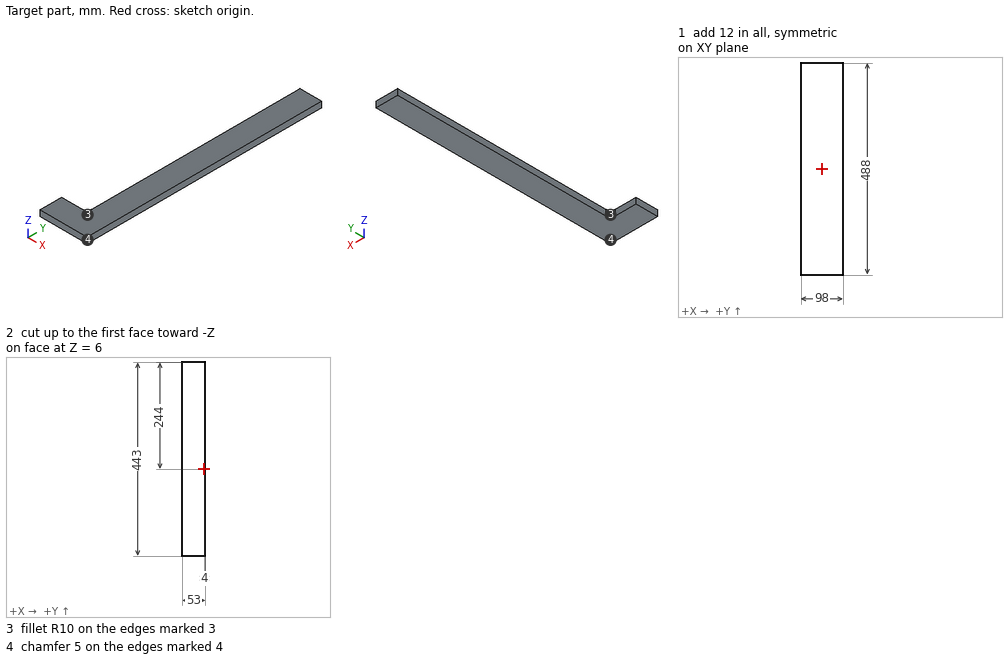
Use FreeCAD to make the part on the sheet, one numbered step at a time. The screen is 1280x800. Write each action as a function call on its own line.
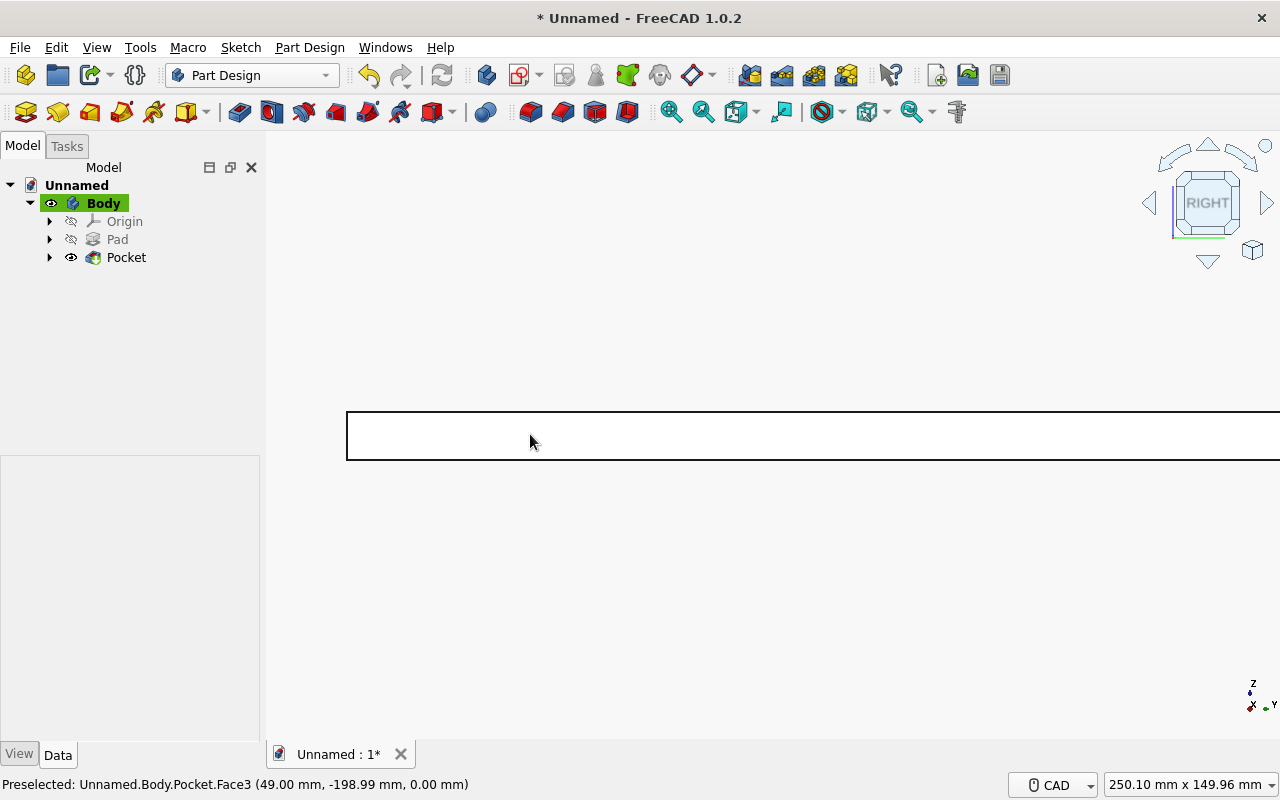
key(v)
key(f)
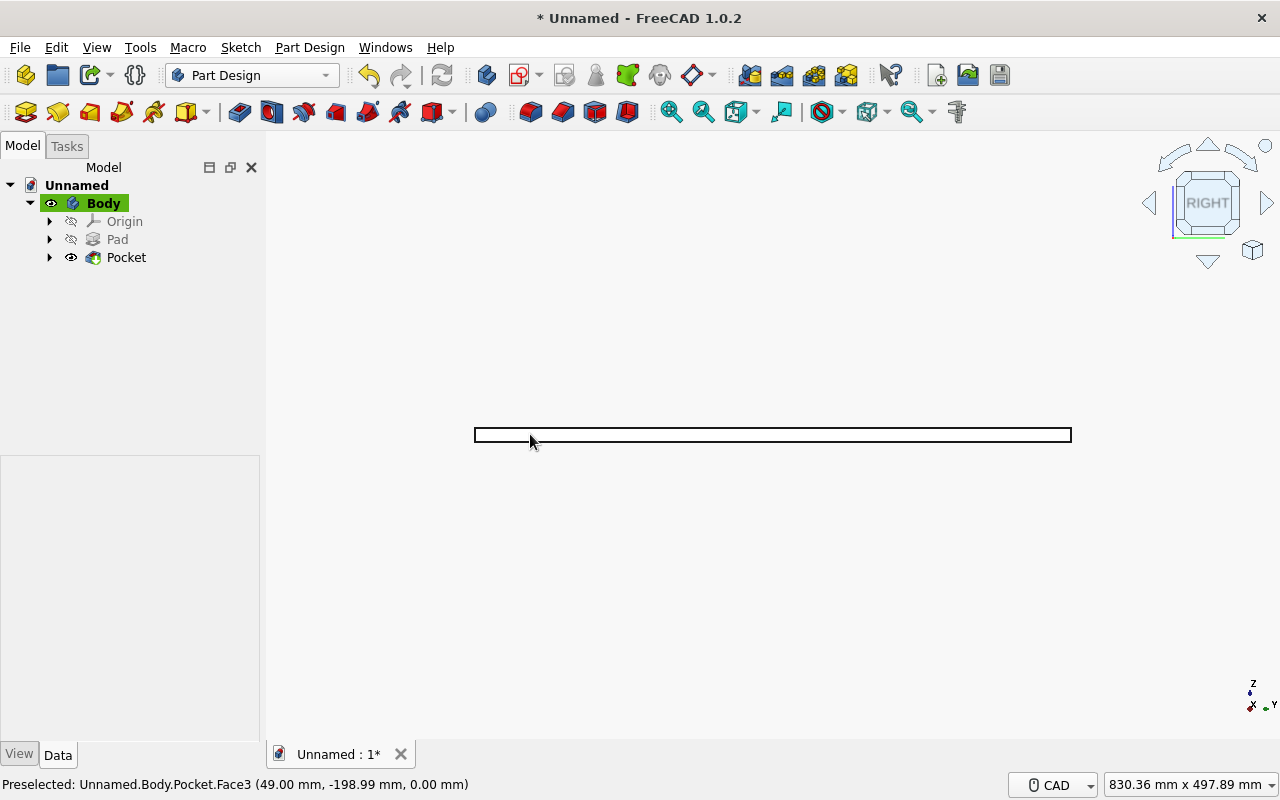
key(5)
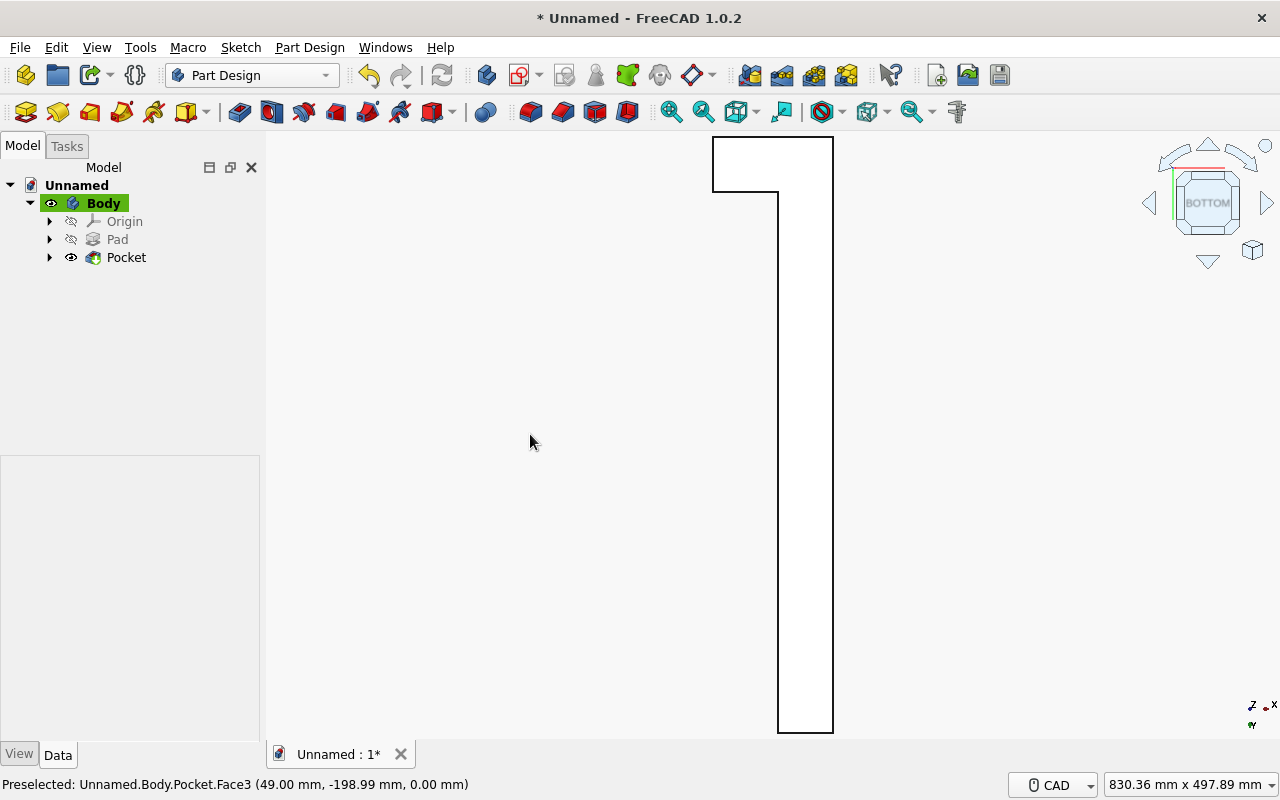
scroll(778, 191, up, 6)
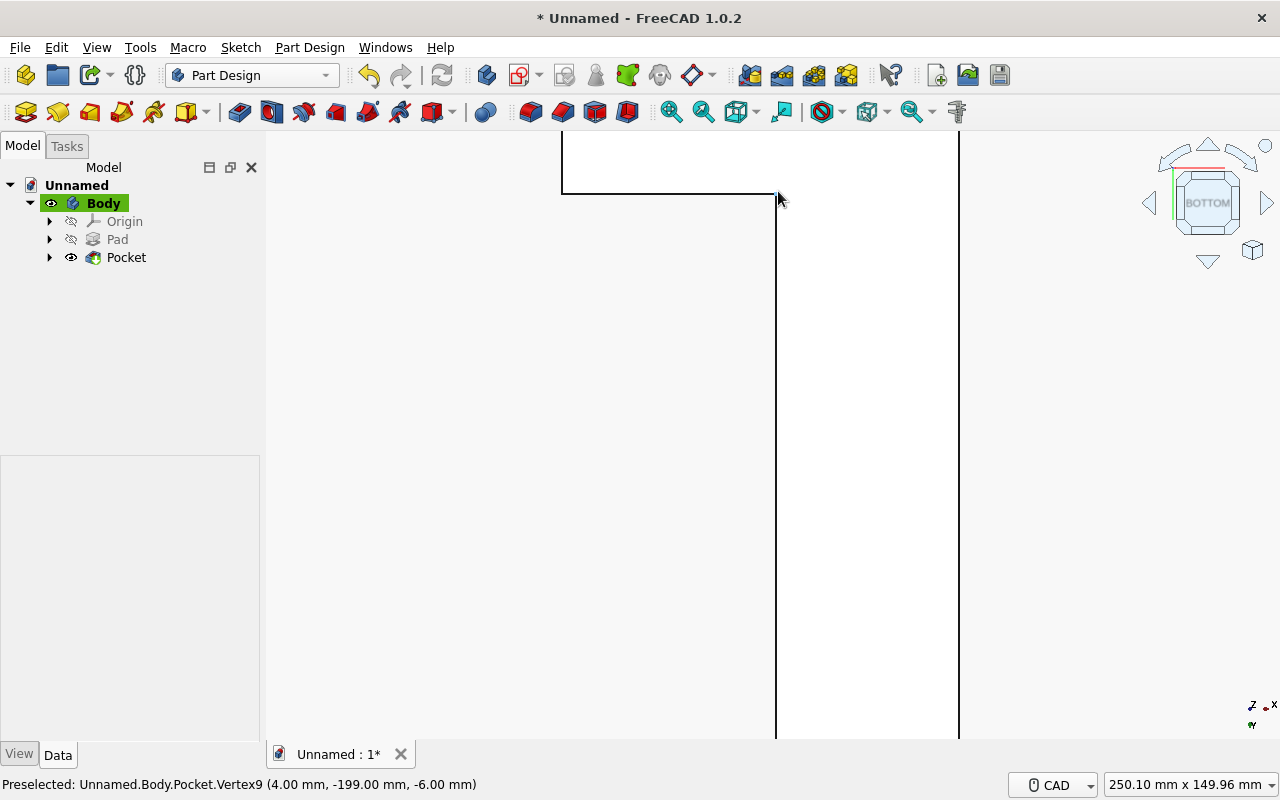
key(v)
key(f)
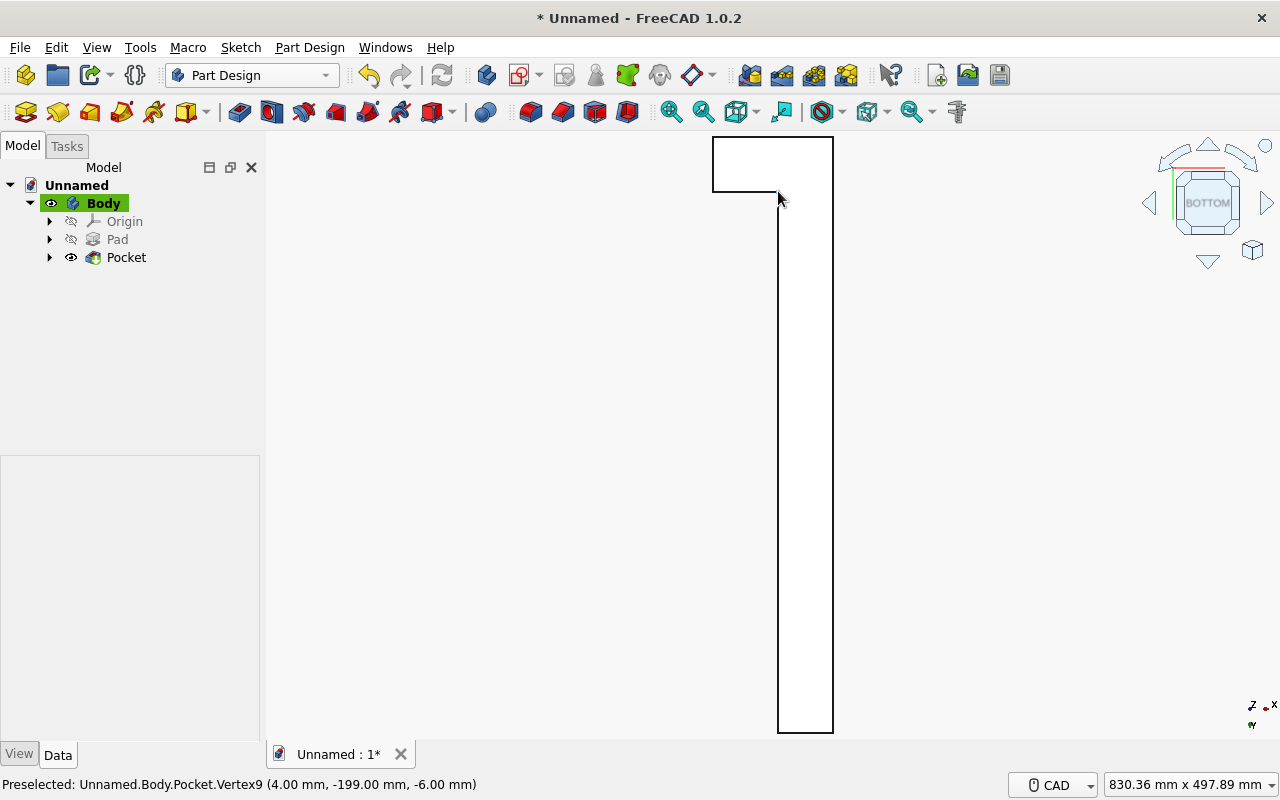
key(4)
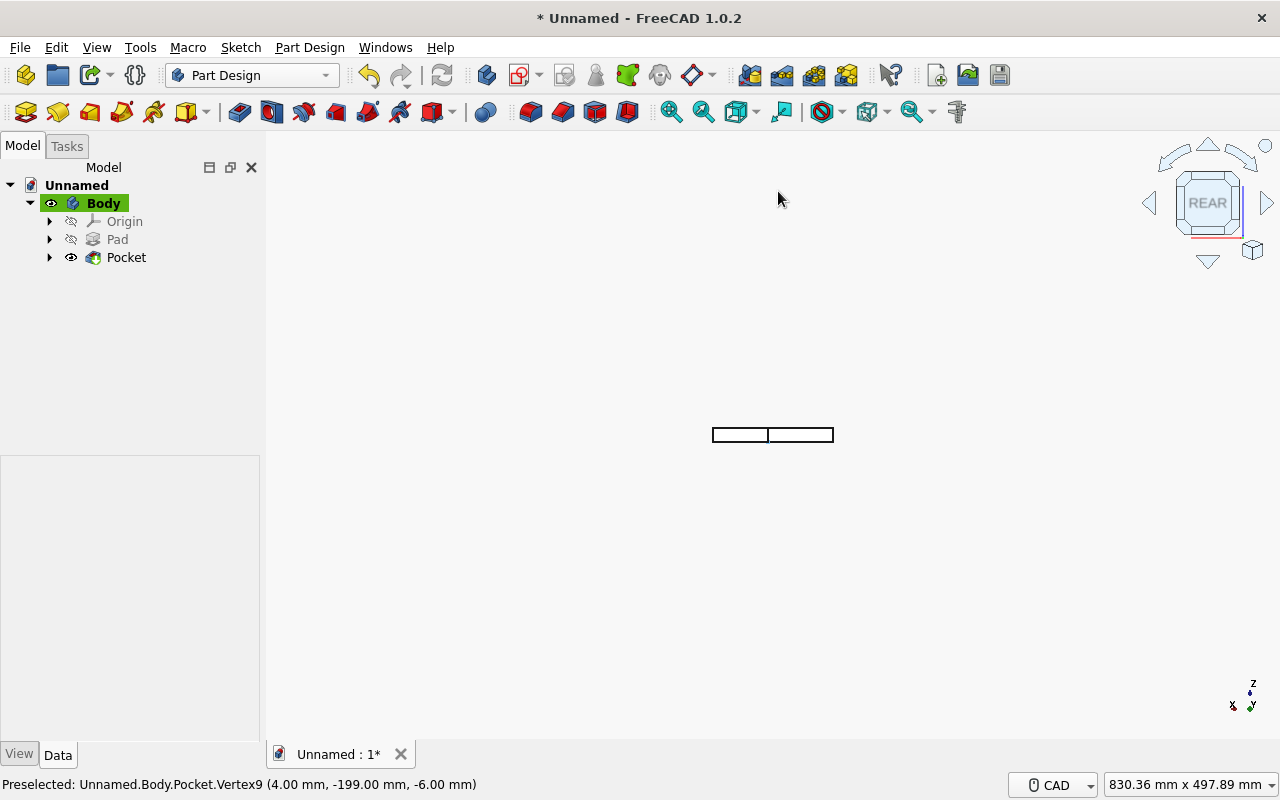
key(v)
key(f)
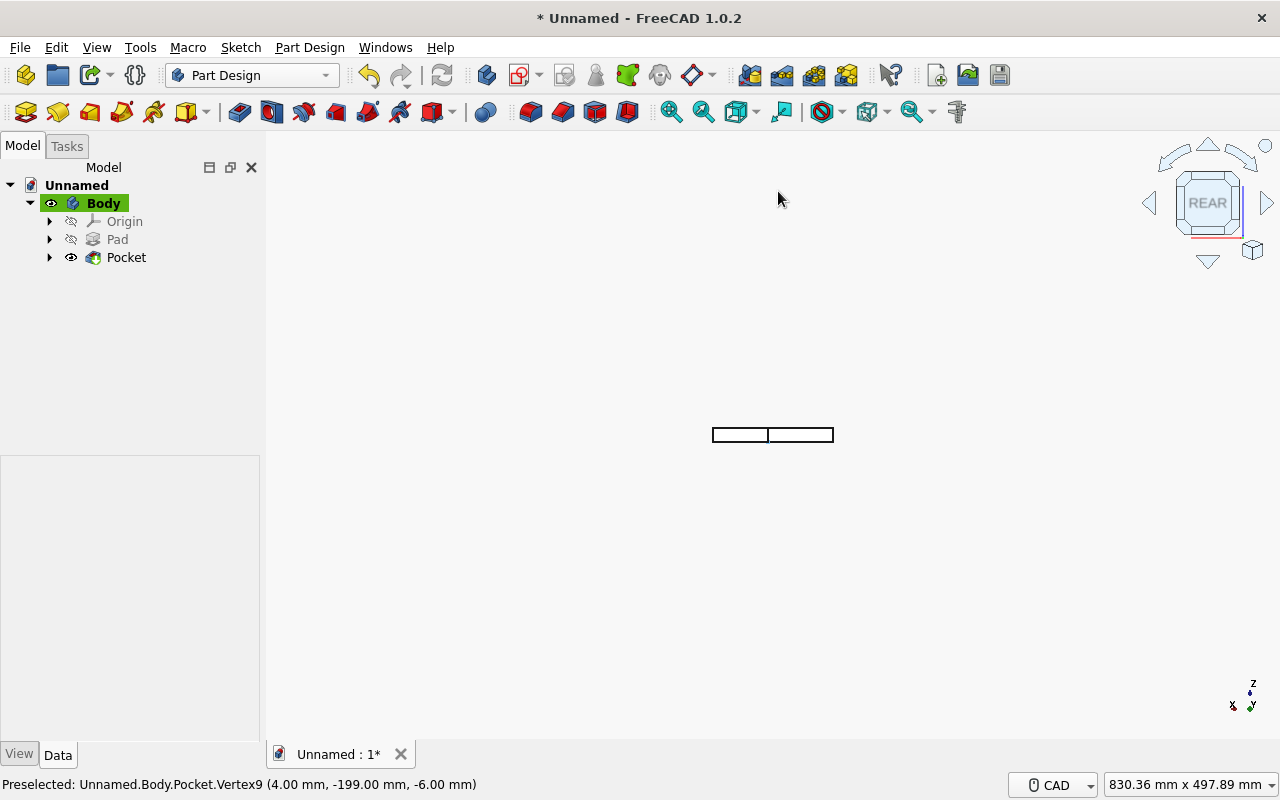
scroll(768, 434, up, 6)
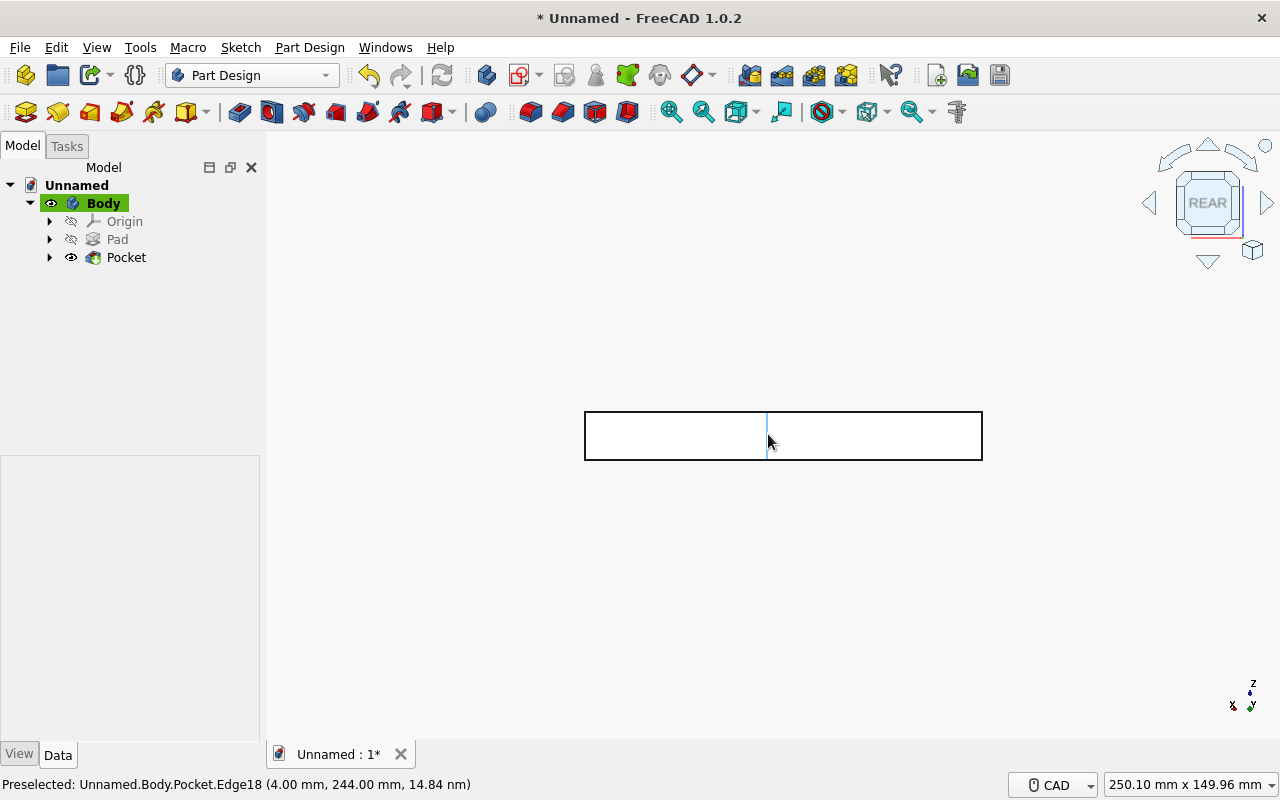
key(v)
key(f)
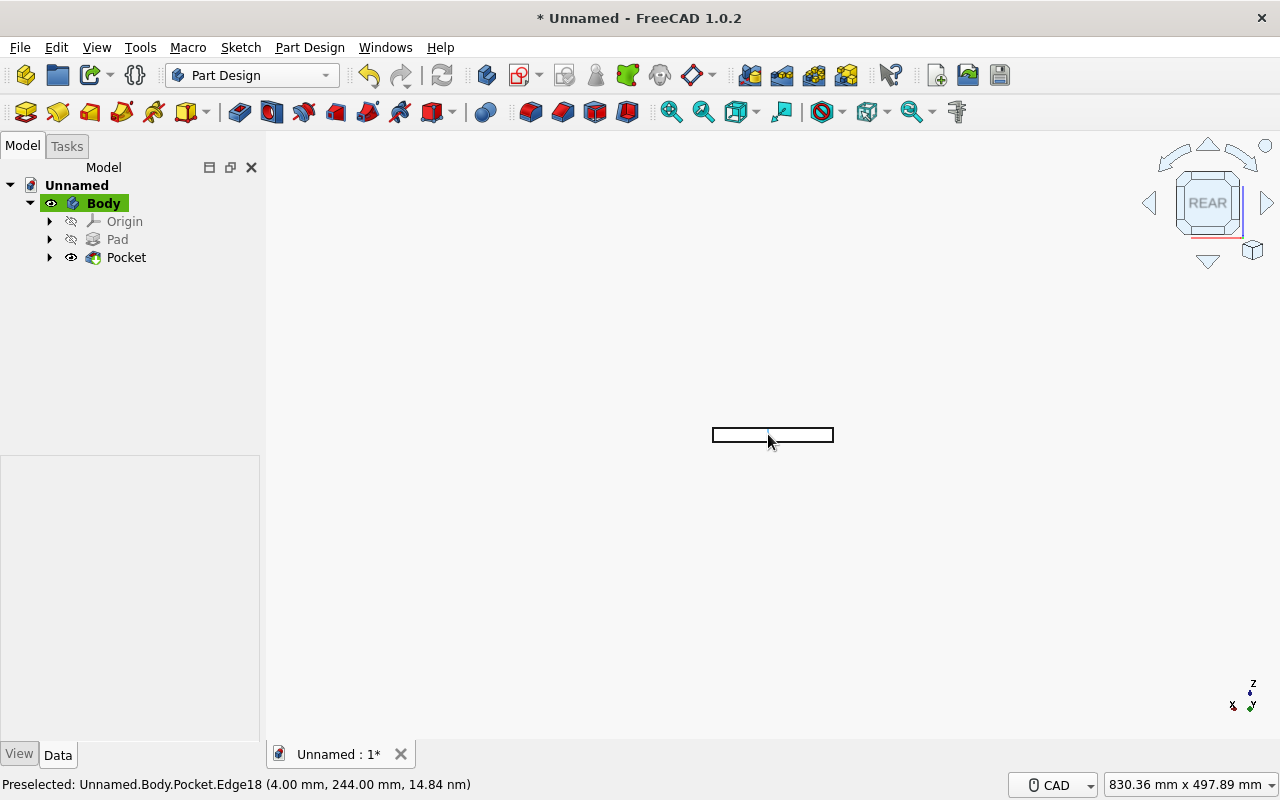
key(6)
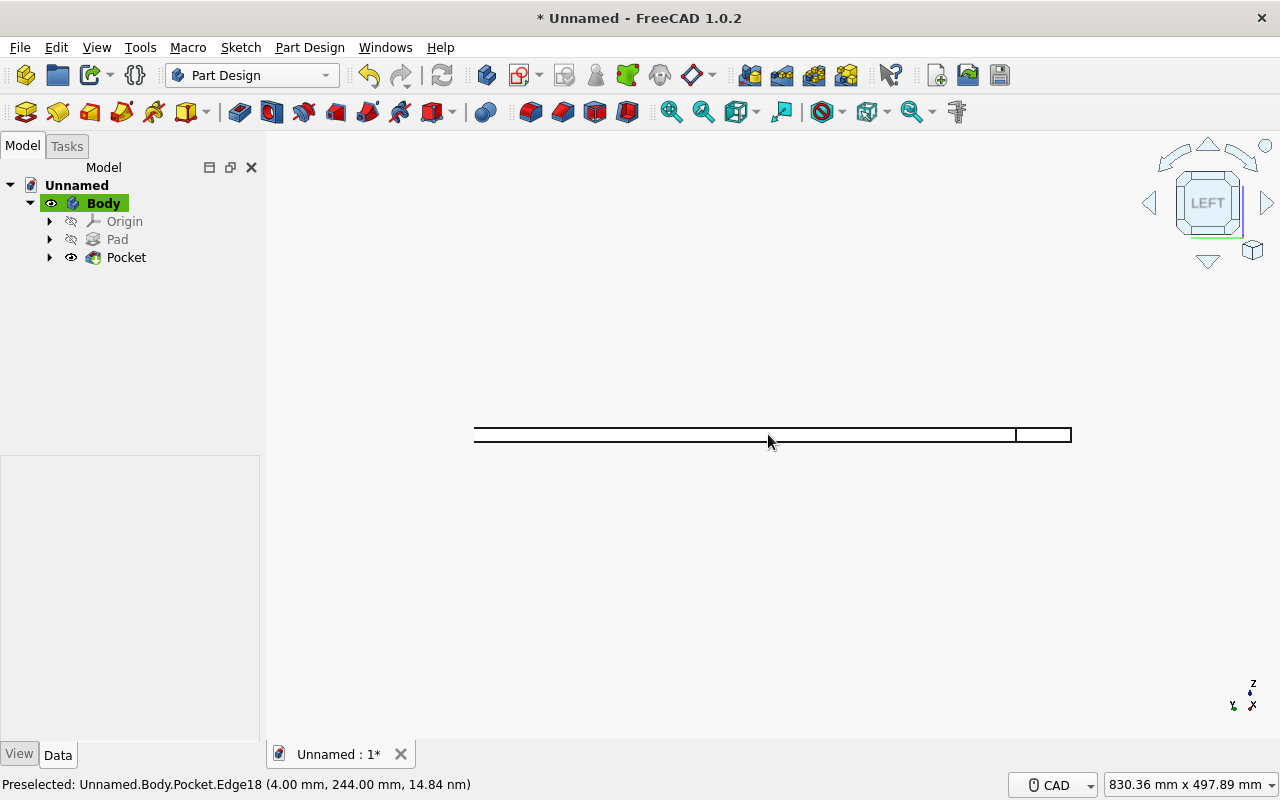
scroll(1016, 434, up, 6)